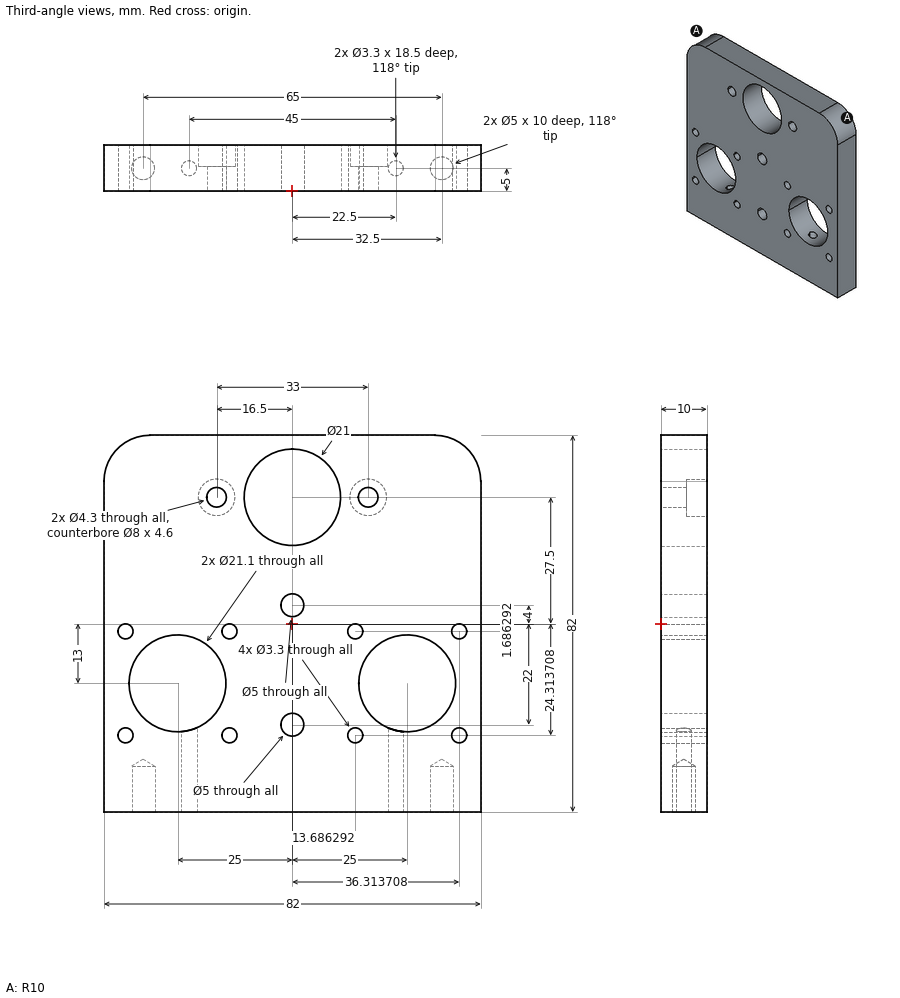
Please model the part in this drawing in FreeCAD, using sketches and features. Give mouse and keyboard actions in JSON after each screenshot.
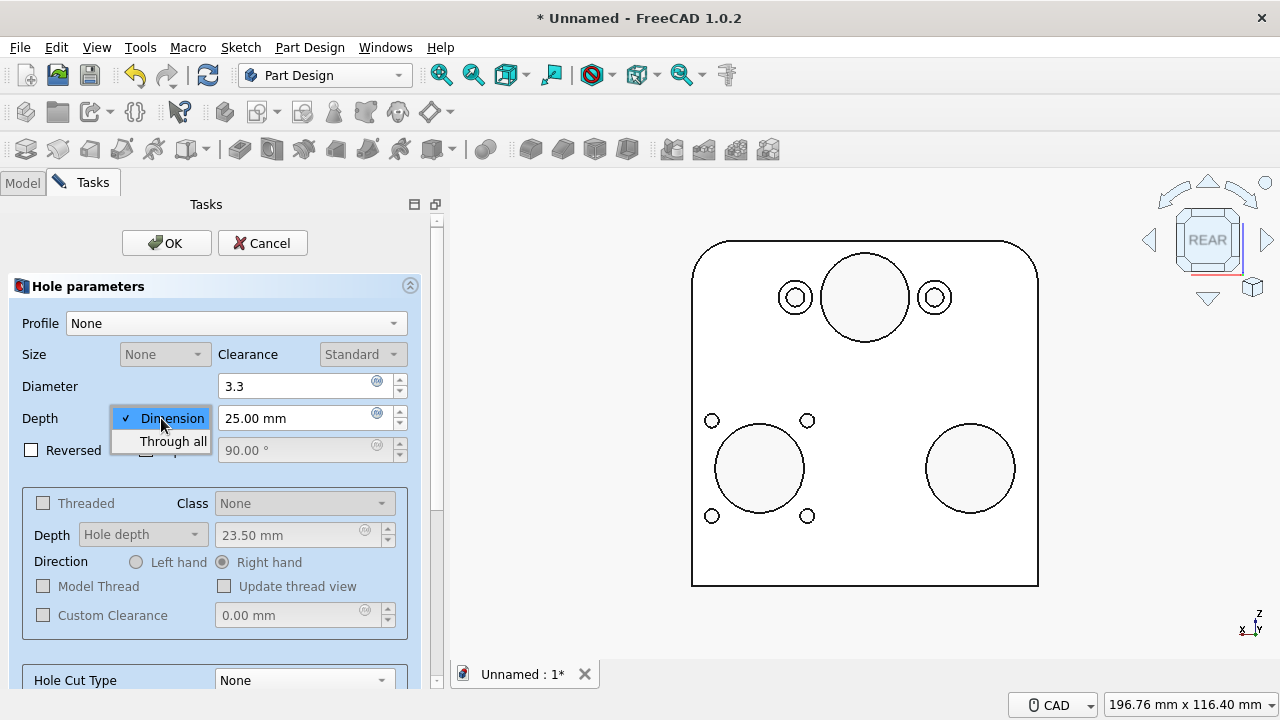
{"action": "left_click", "coordinate": [160, 442]}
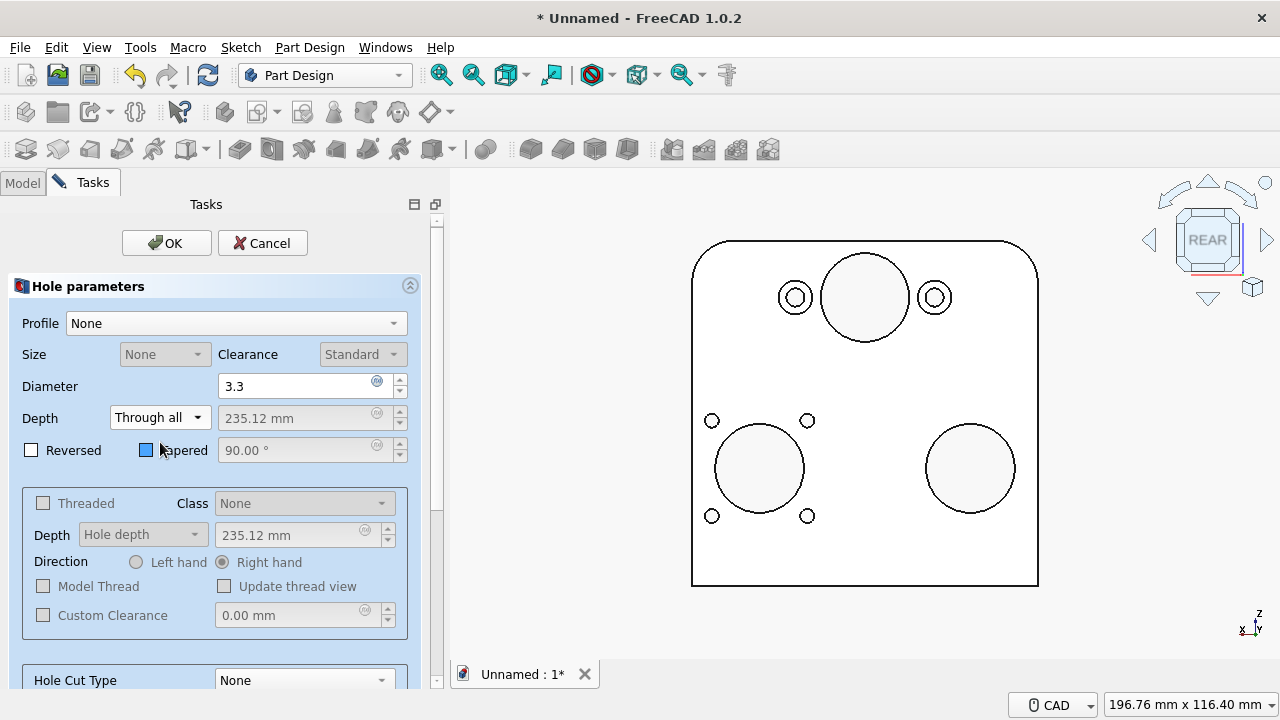
{"action": "left_click", "coordinate": [167, 243]}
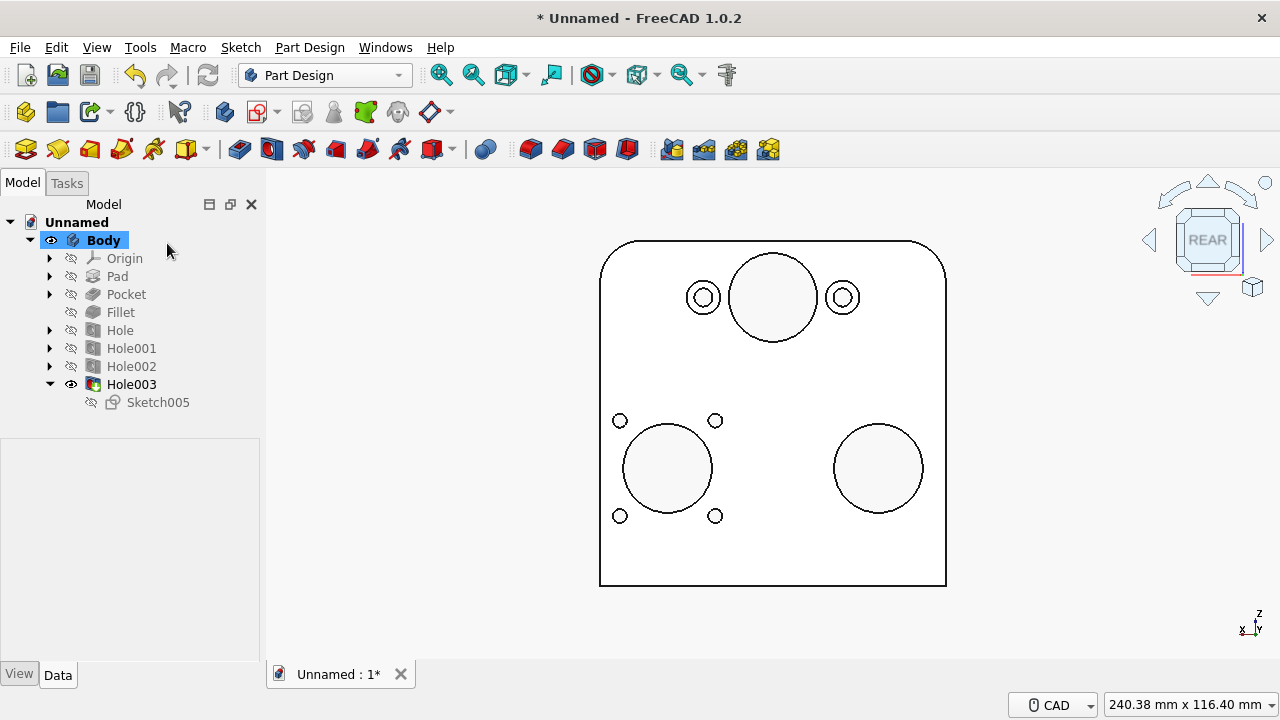
{"action": "left_click", "coordinate": [116, 384]}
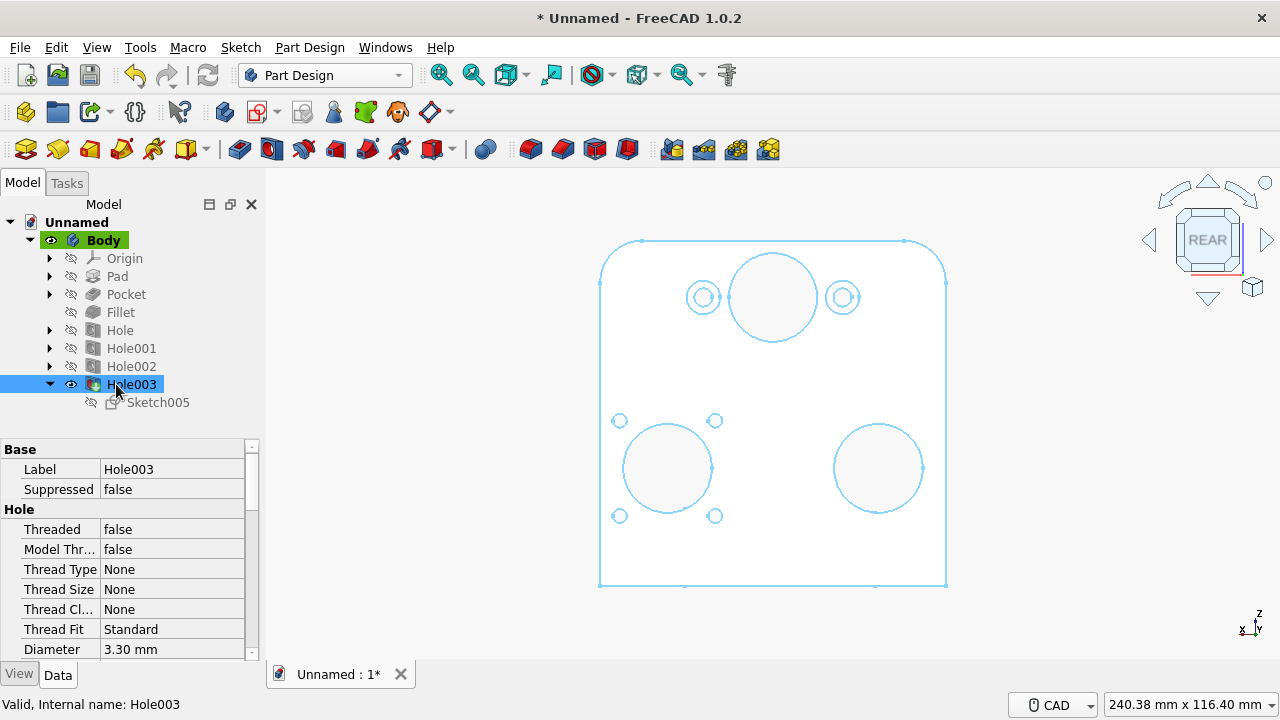
{"action": "left_click", "coordinate": [672, 150]}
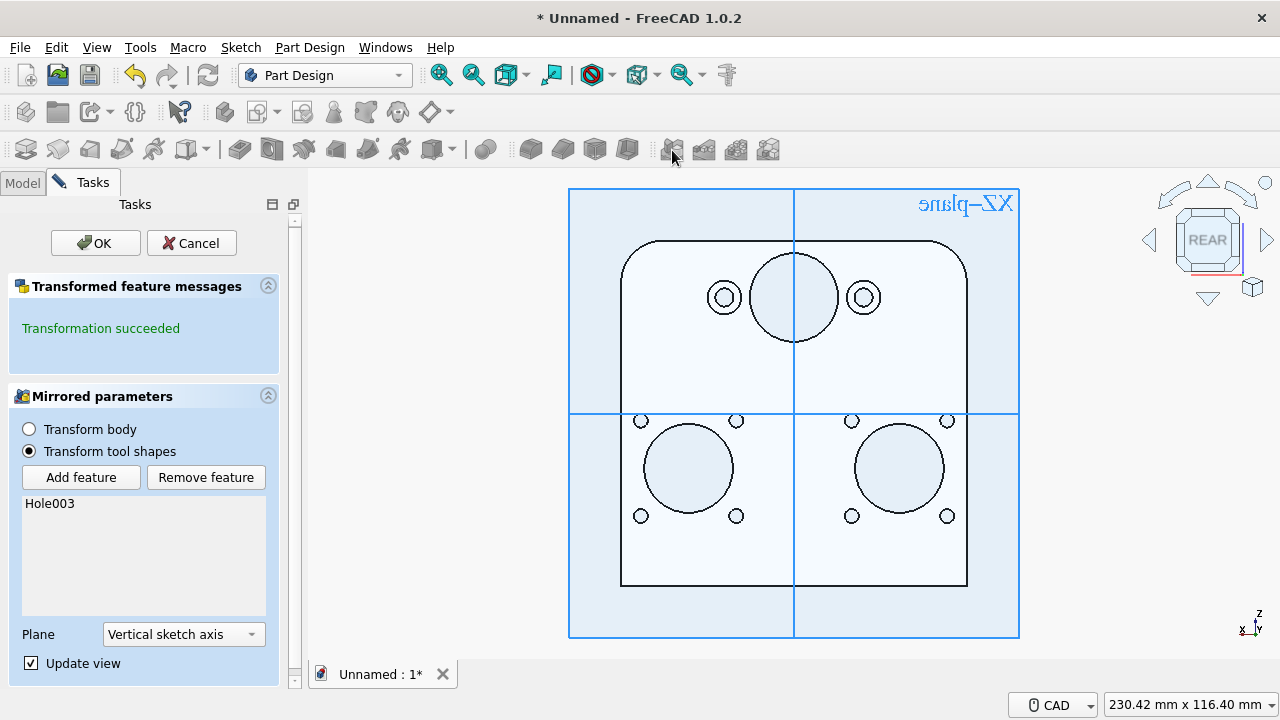
{"action": "left_click", "coordinate": [184, 634]}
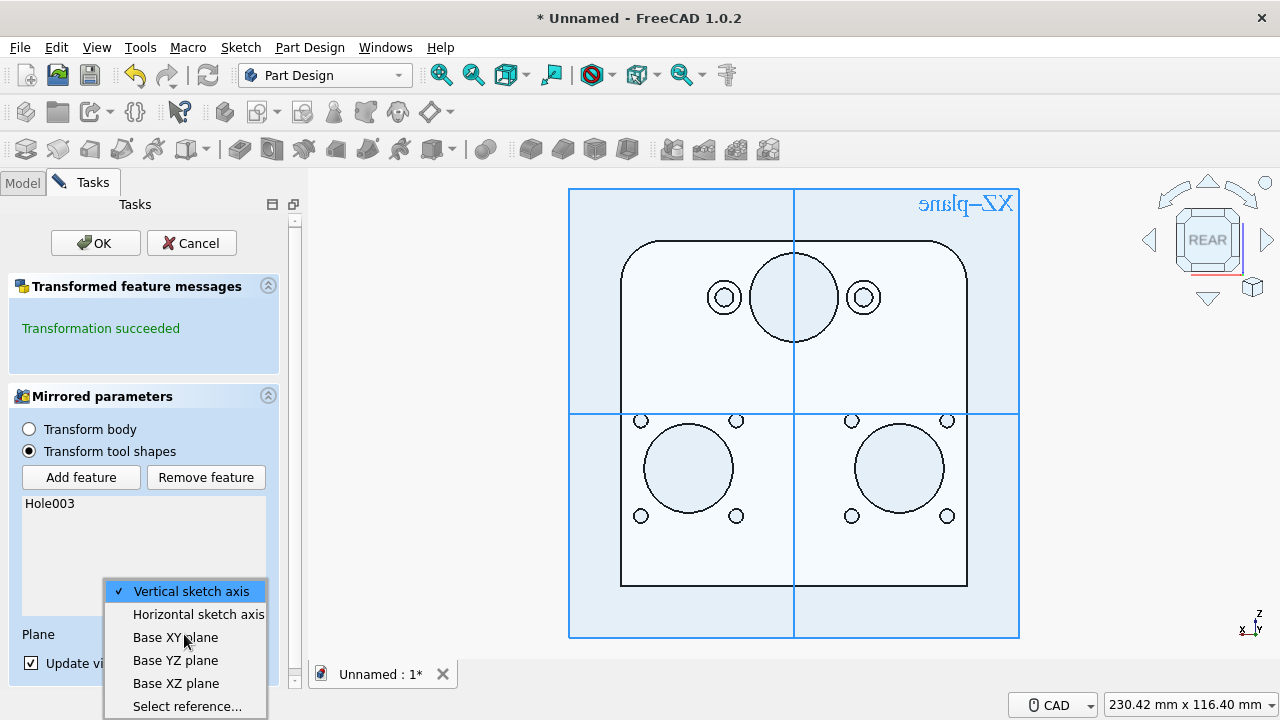
{"action": "left_click", "coordinate": [184, 660]}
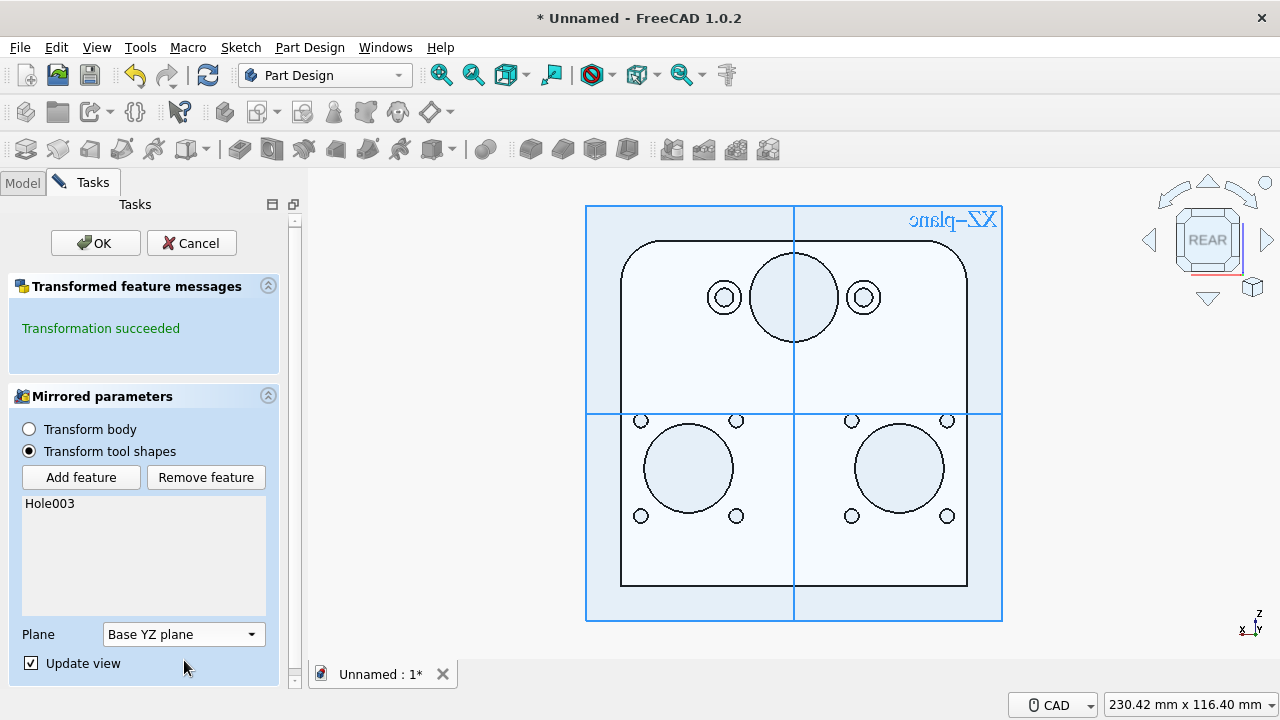
{"action": "left_click", "coordinate": [96, 243]}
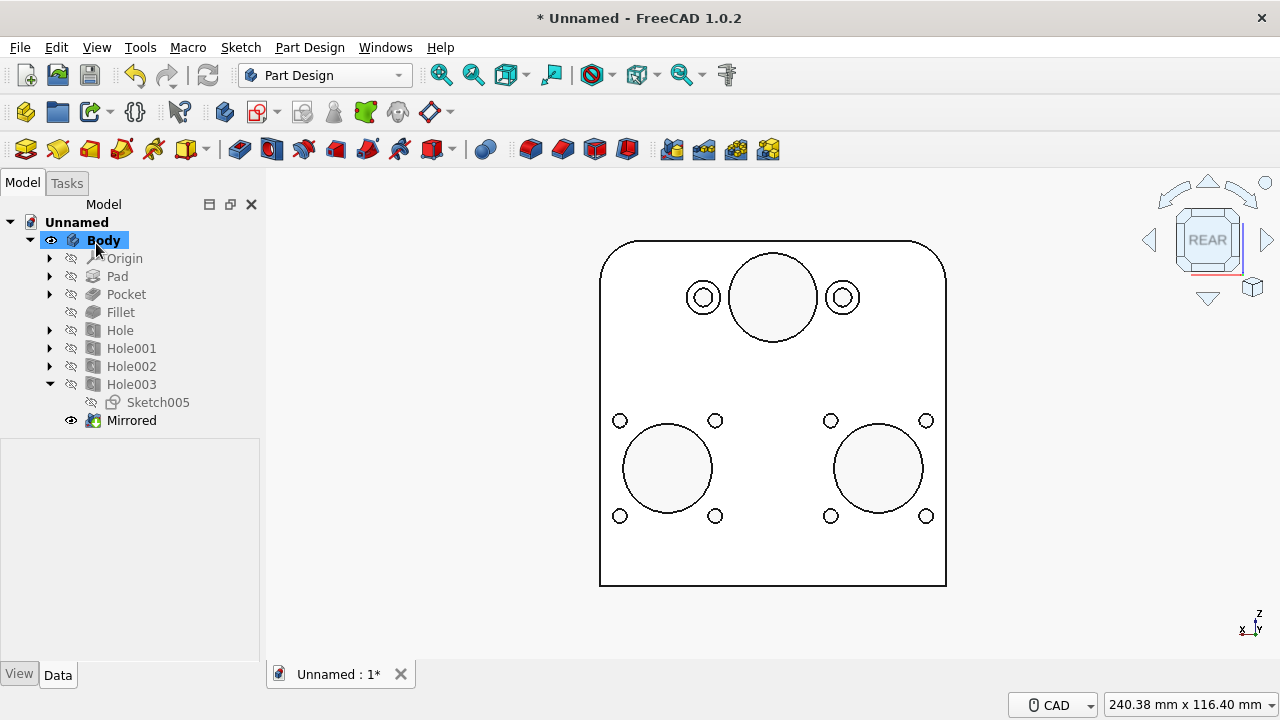
{"action": "left_click", "coordinate": [773, 462]}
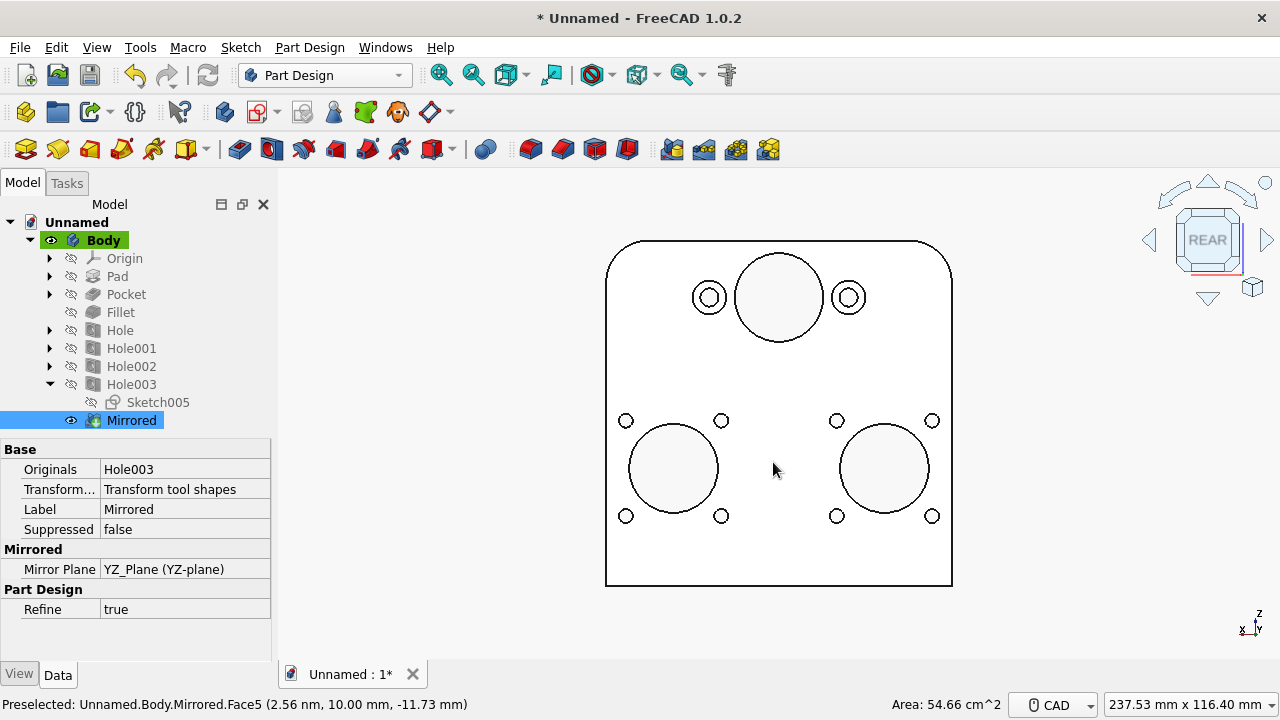
{"action": "left_click", "coordinate": [258, 112]}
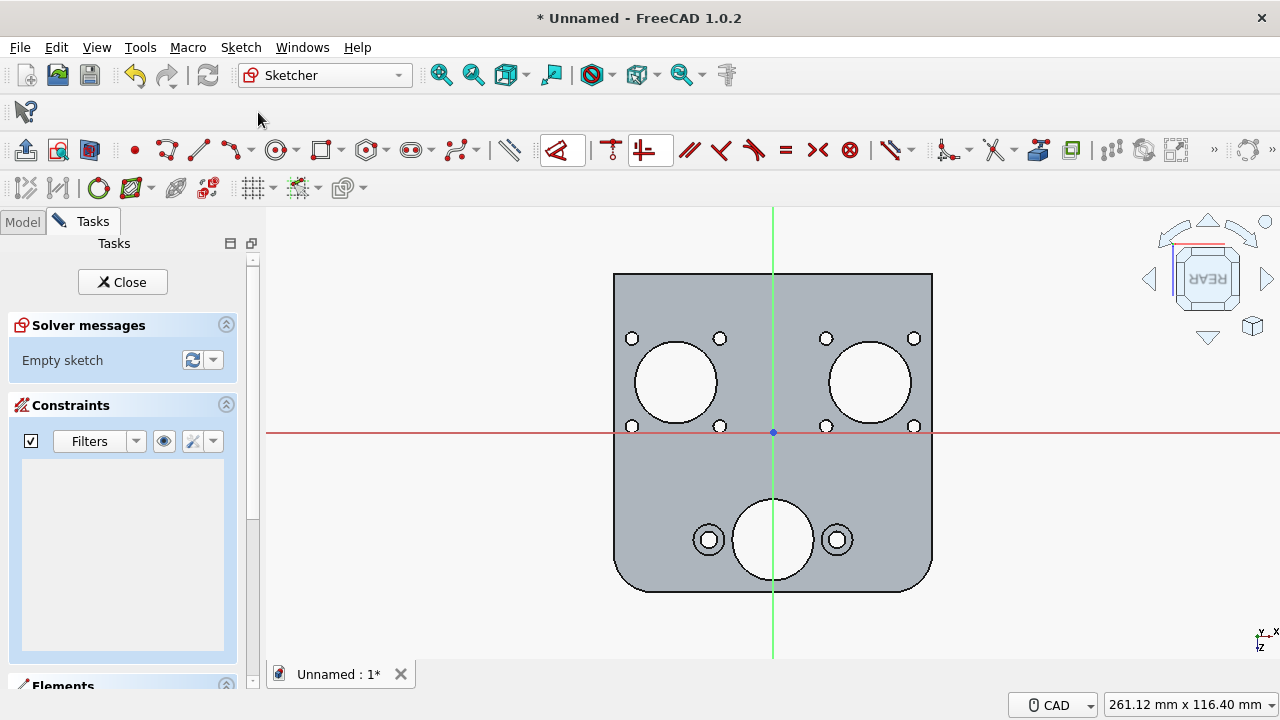
{"action": "scroll", "coordinate": [778, 341], "scroll_direction": "up", "scroll_amount": 13}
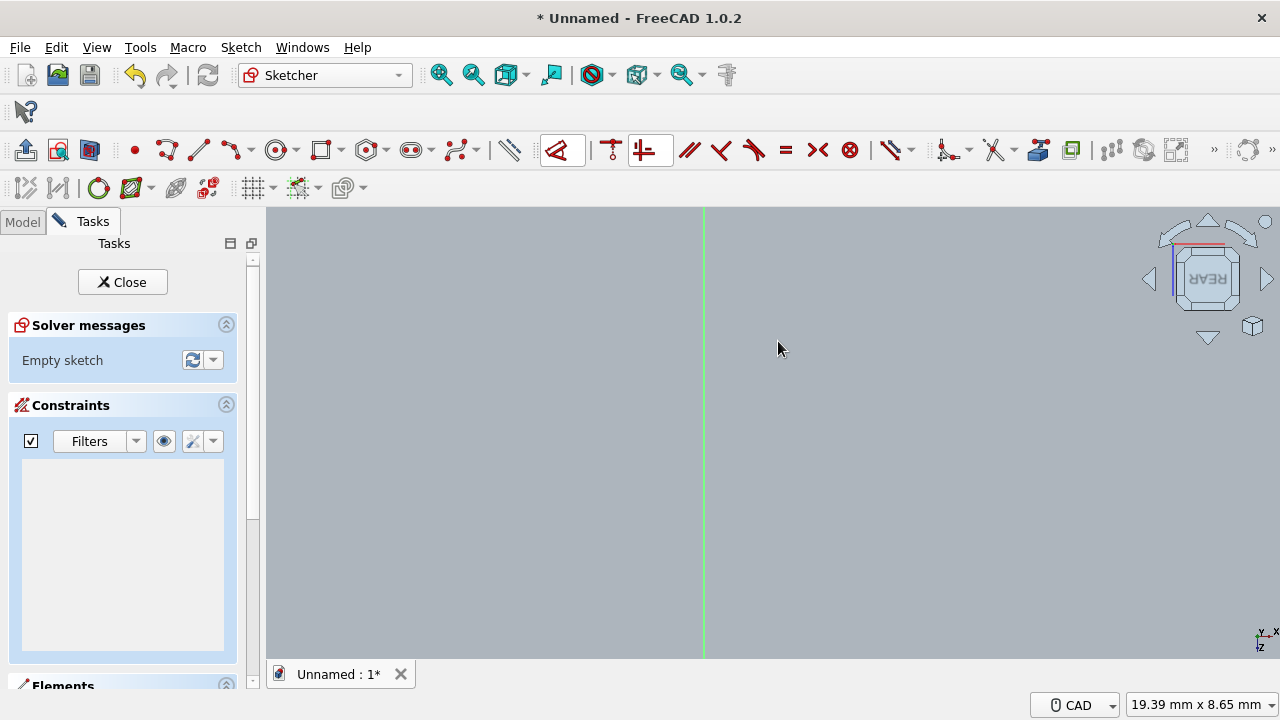
{"action": "left_click", "coordinate": [276, 150]}